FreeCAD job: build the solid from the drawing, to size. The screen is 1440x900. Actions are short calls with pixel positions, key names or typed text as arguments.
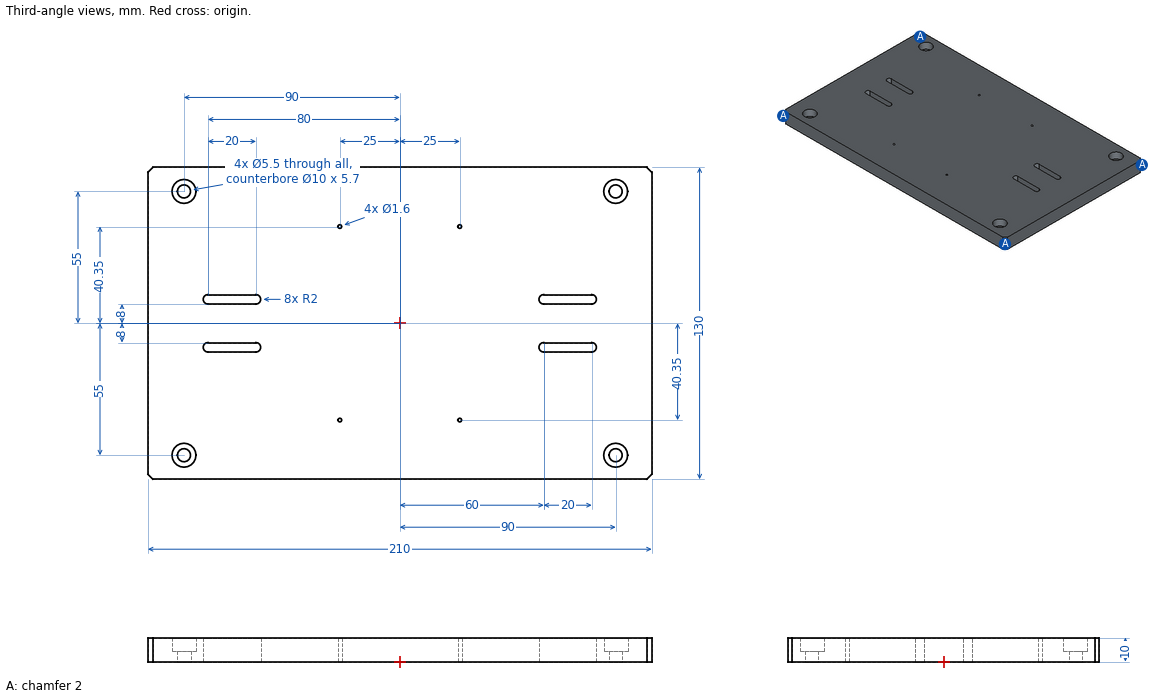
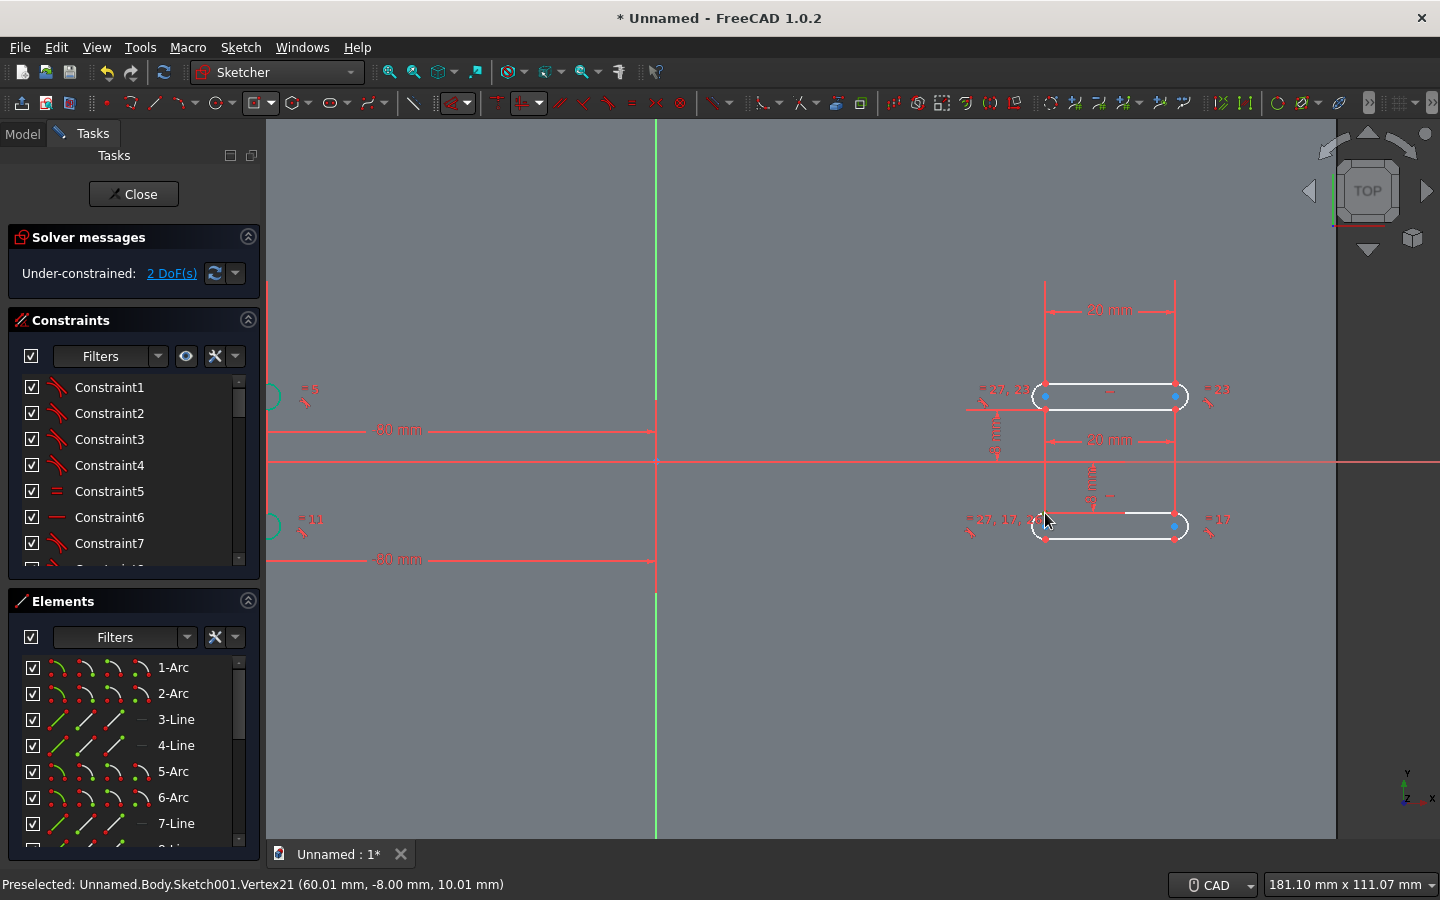
key(l)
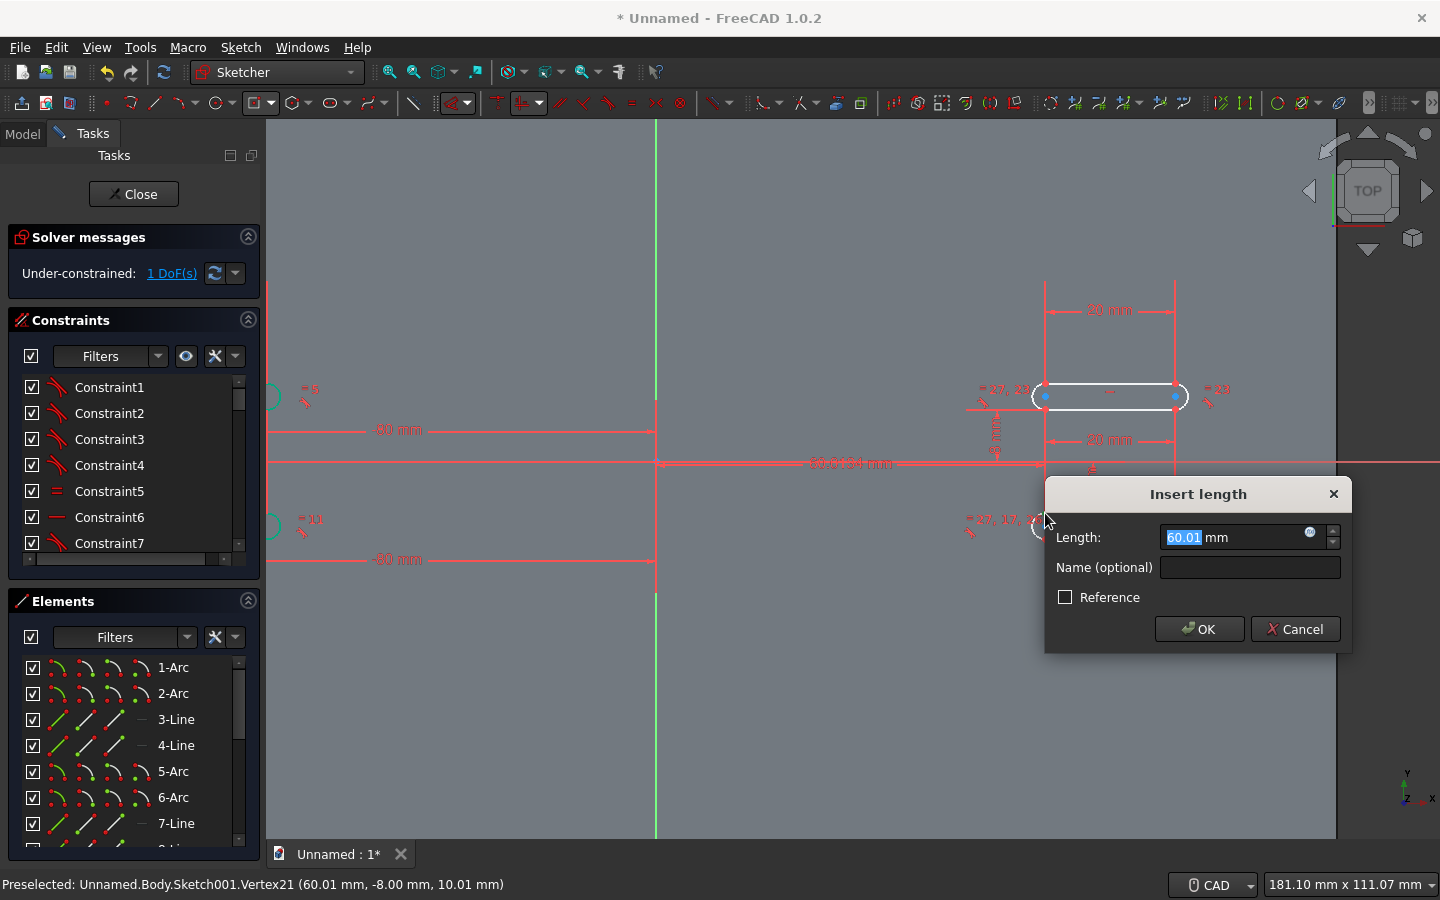
text(60)
key(Return)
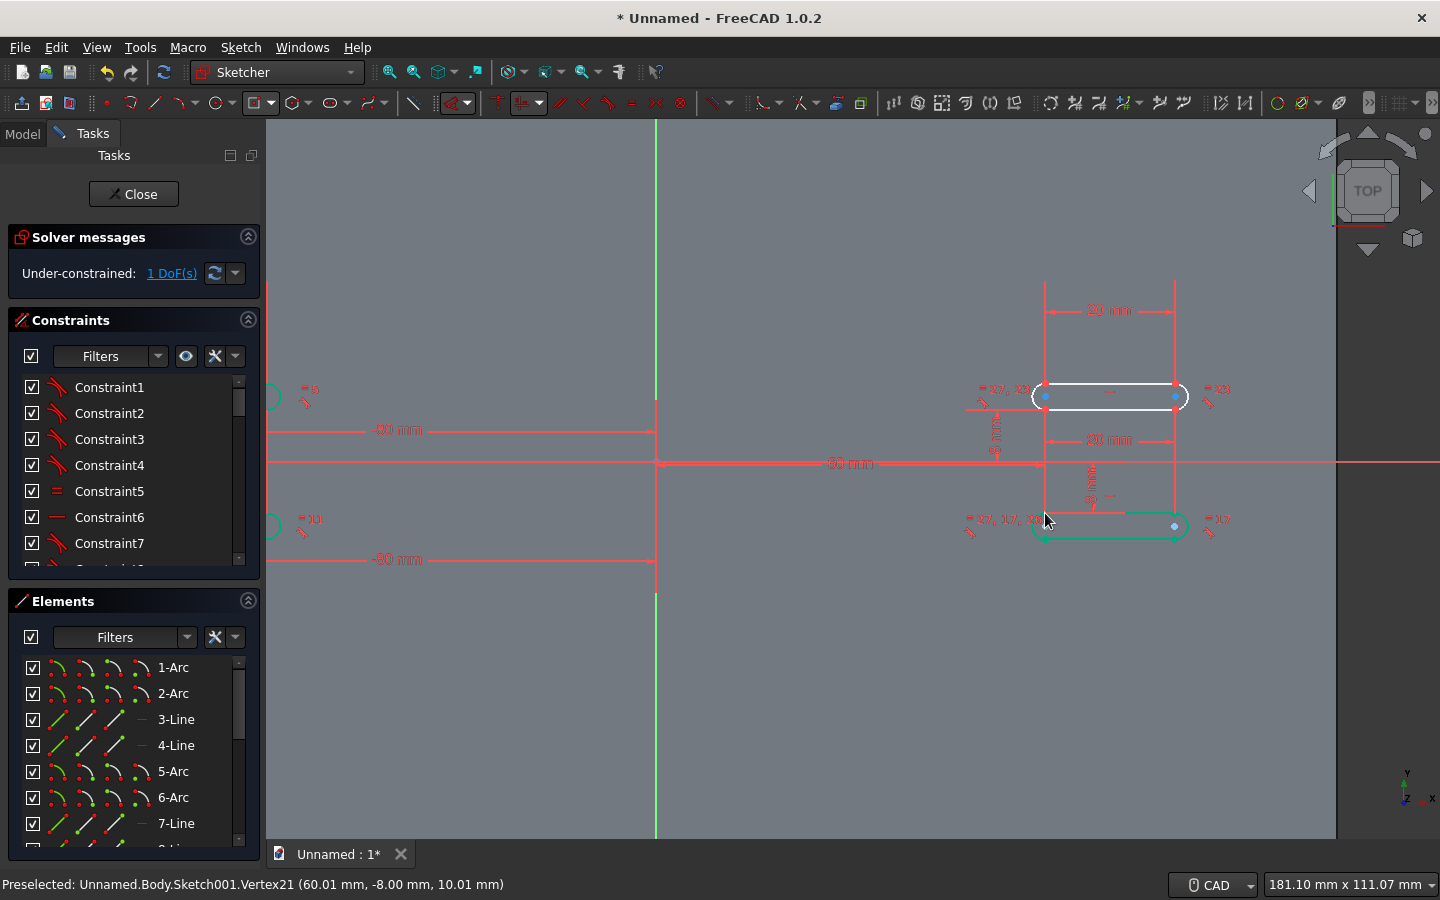
click(1045, 384)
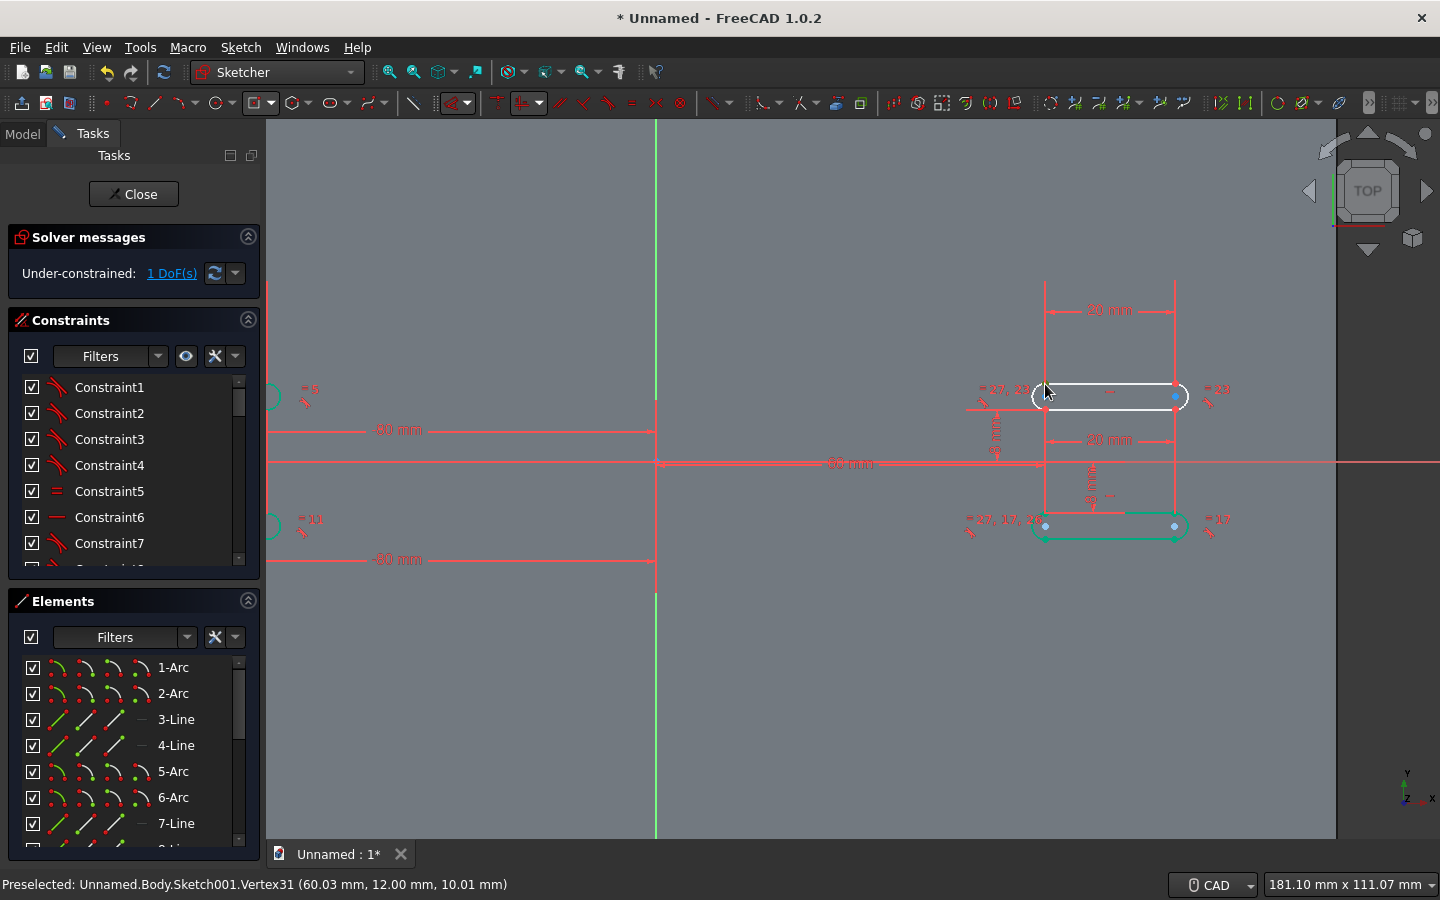
click(470, 104)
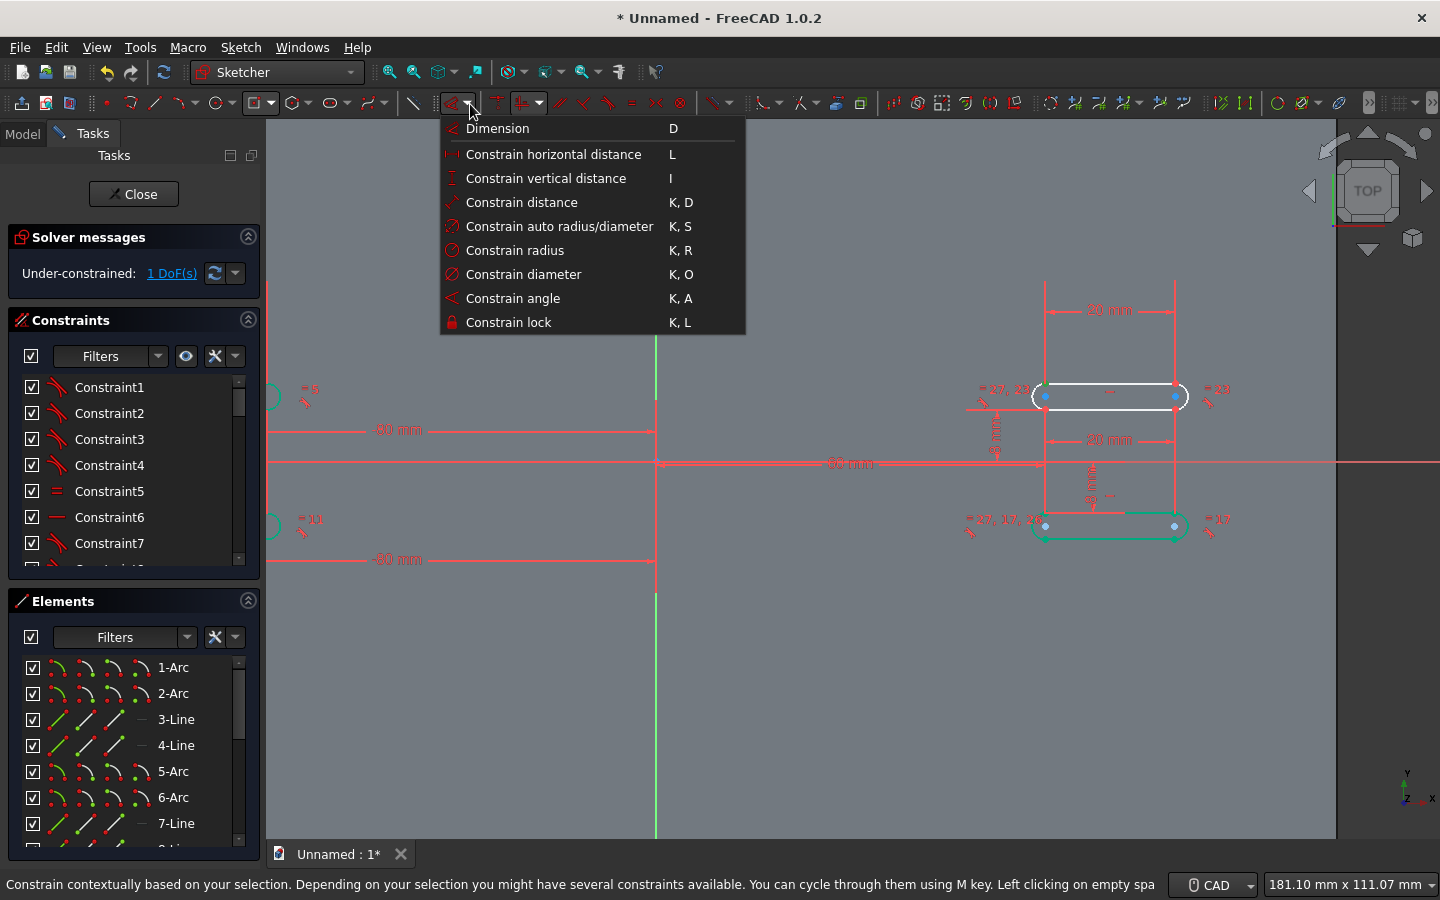
click(593, 154)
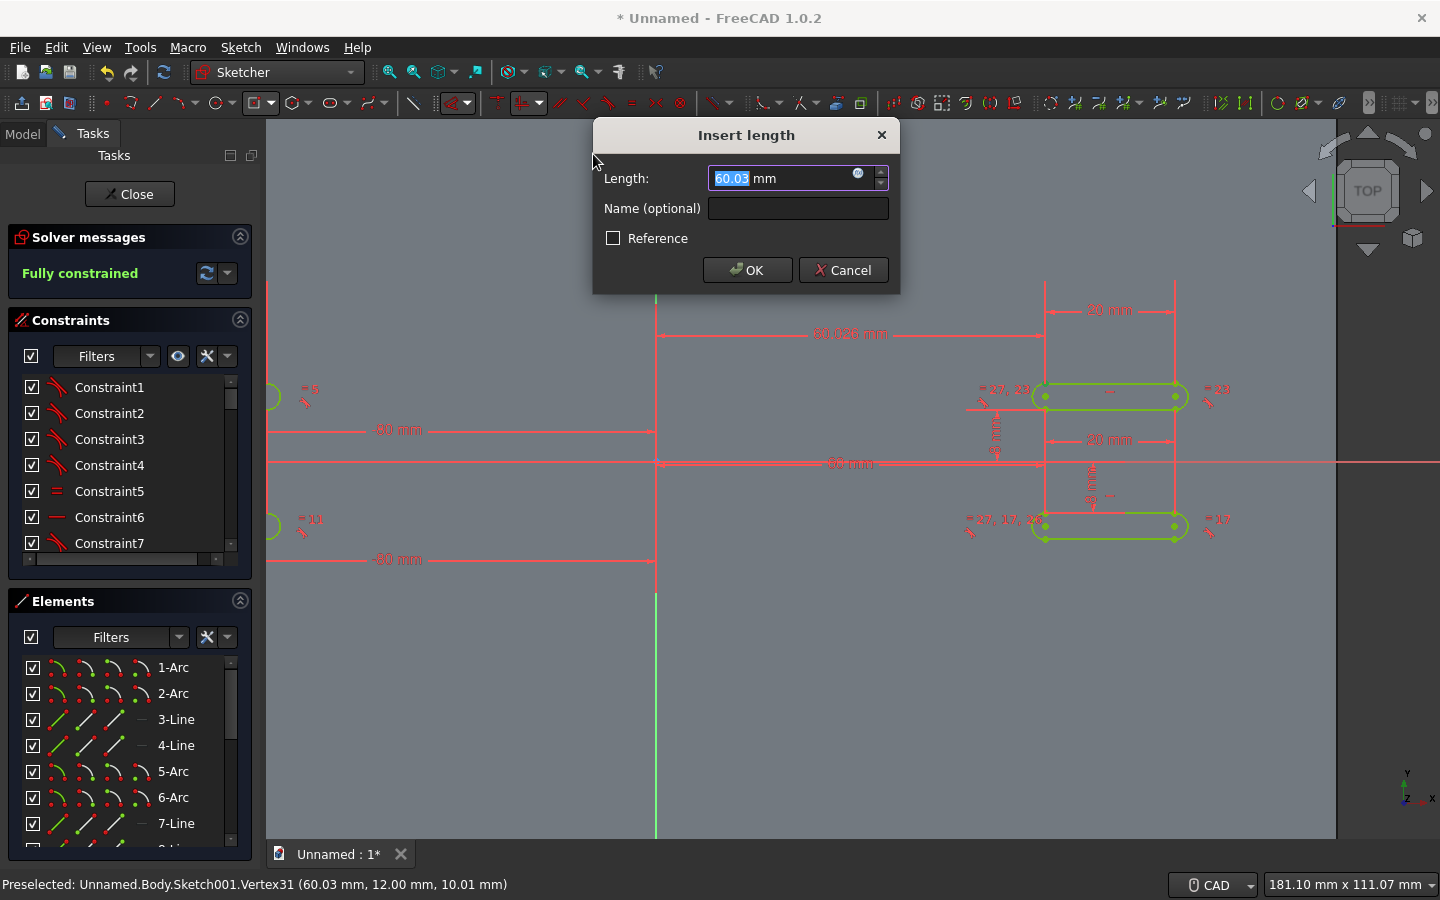
text(60)
key(Return)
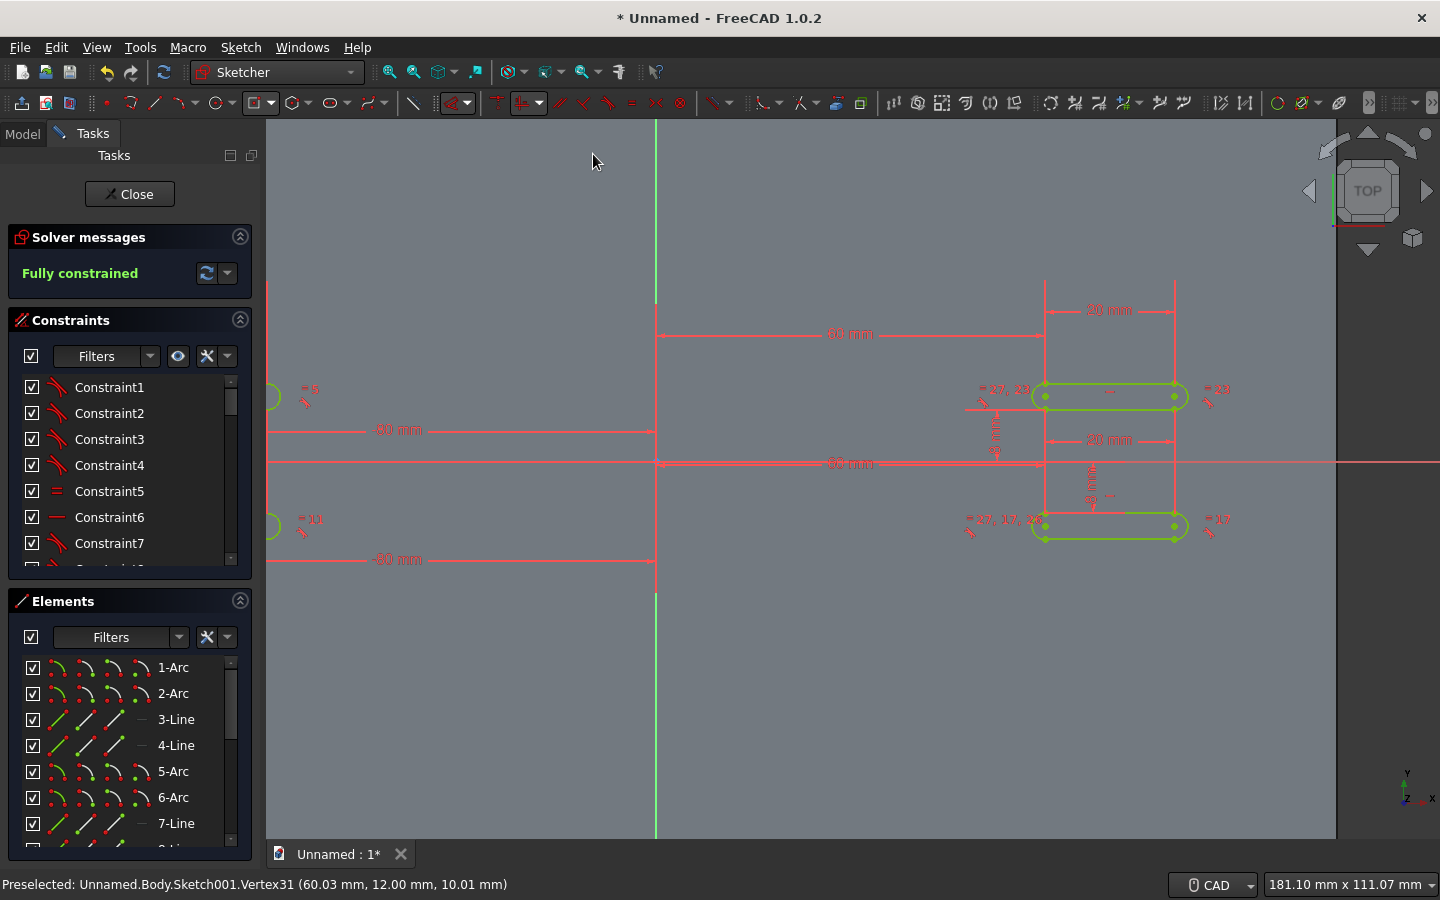
click(130, 194)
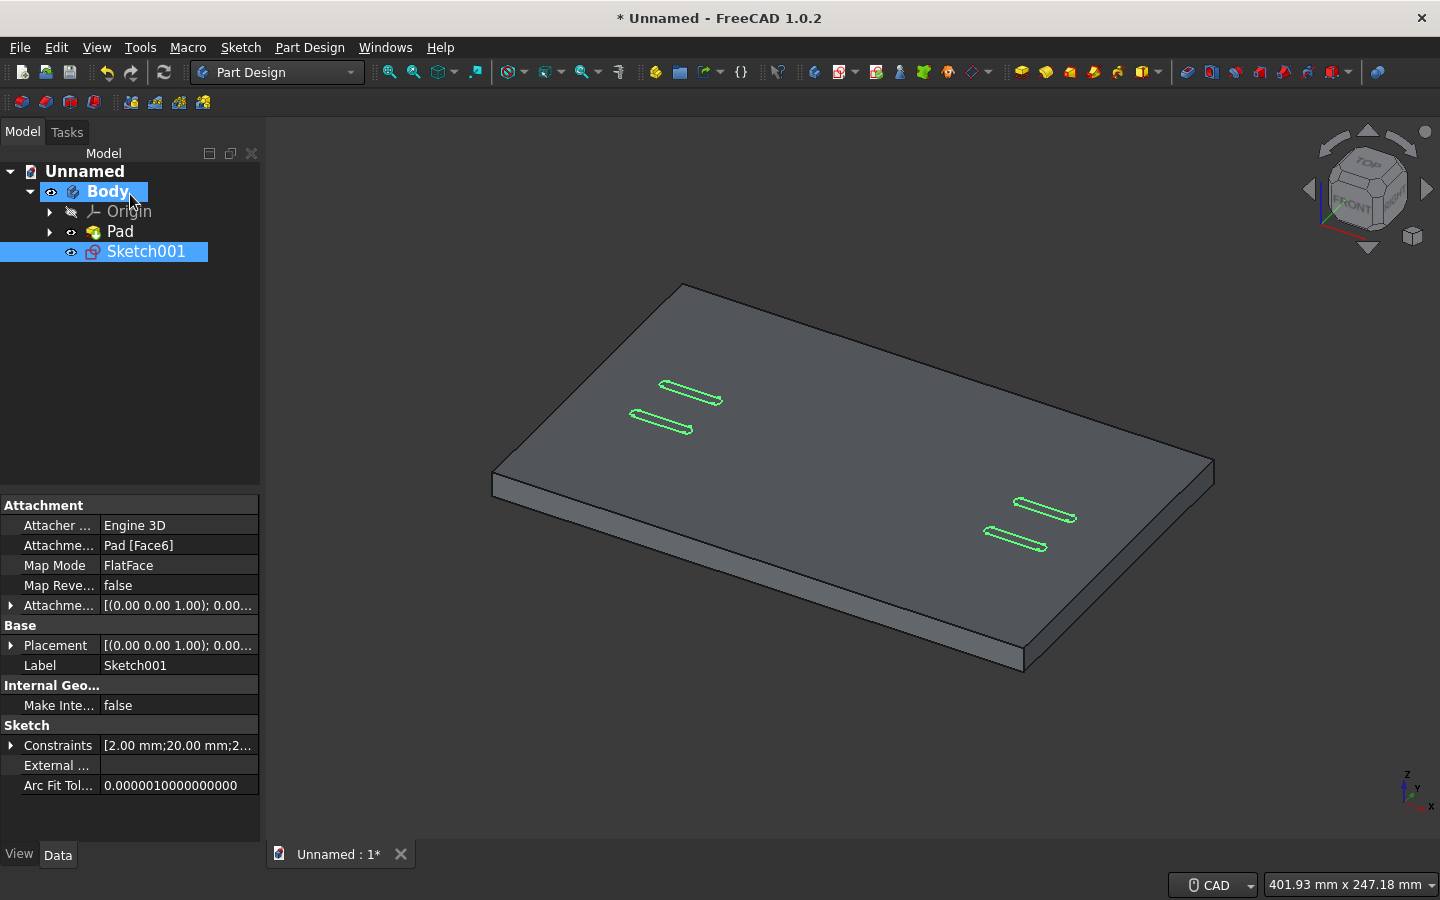
click(1188, 72)